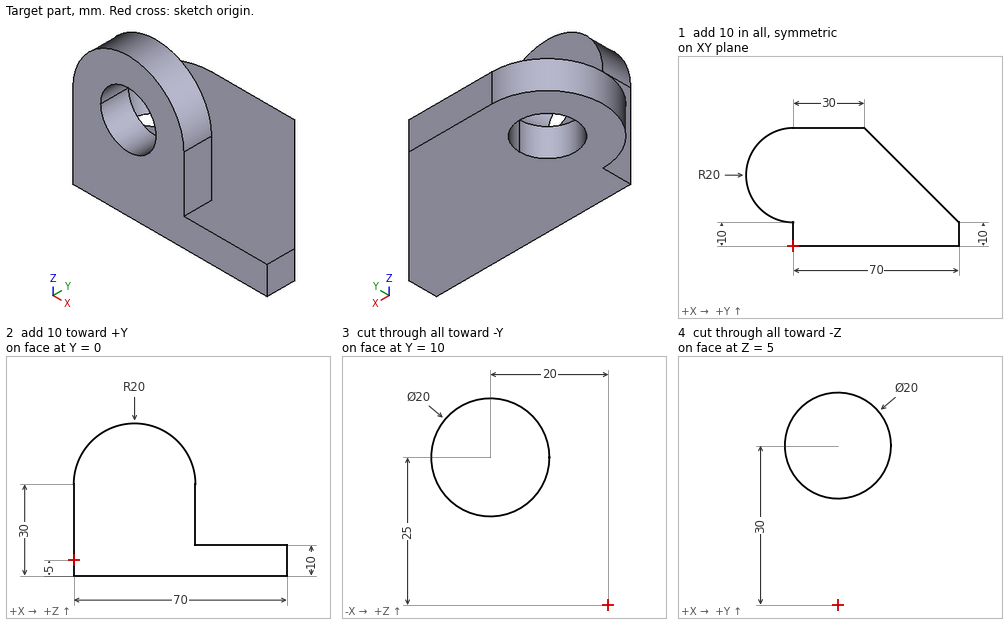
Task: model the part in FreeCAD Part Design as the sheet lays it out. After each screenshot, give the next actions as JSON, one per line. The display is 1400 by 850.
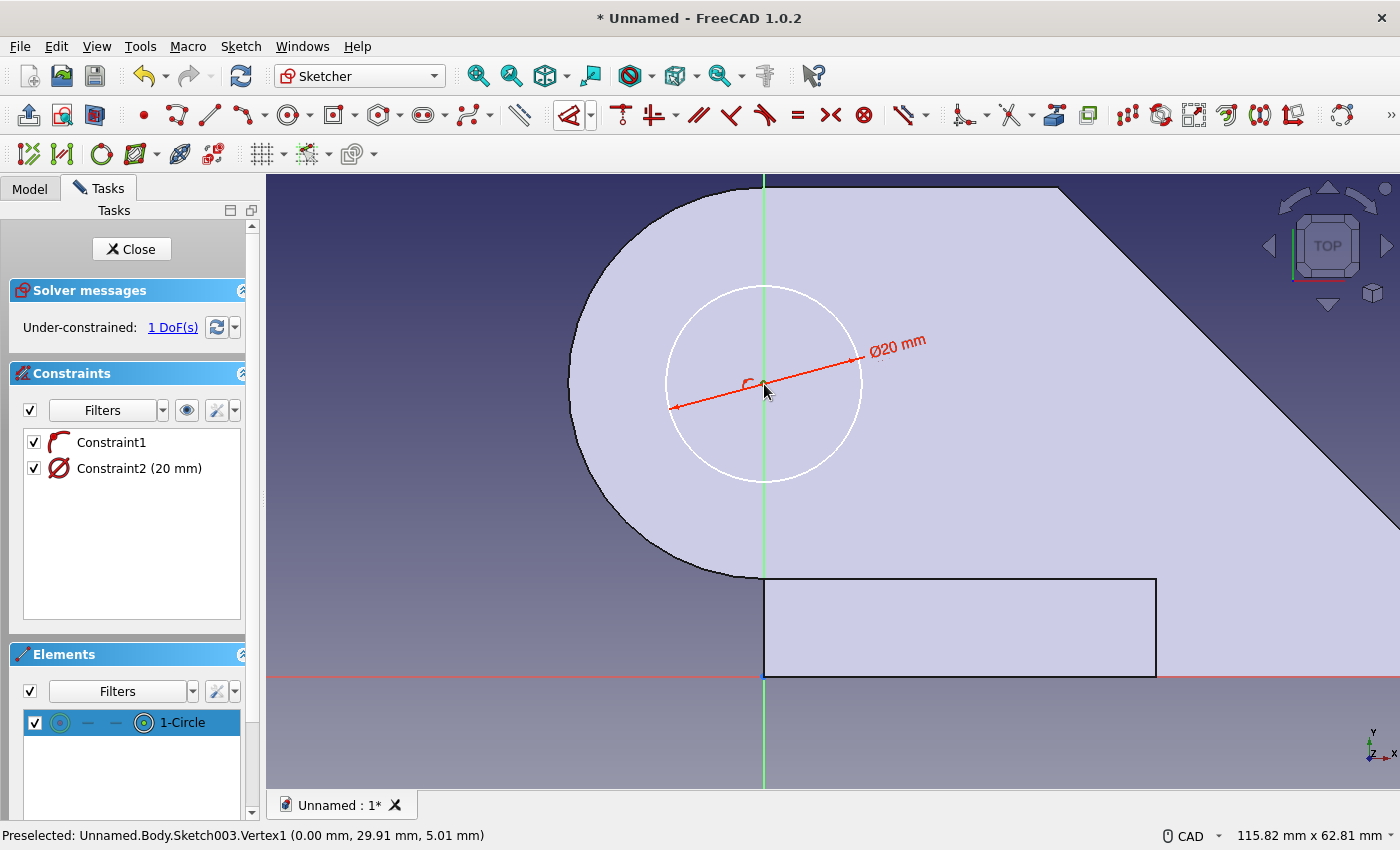
{"action": "left_click", "coordinate": [590, 116]}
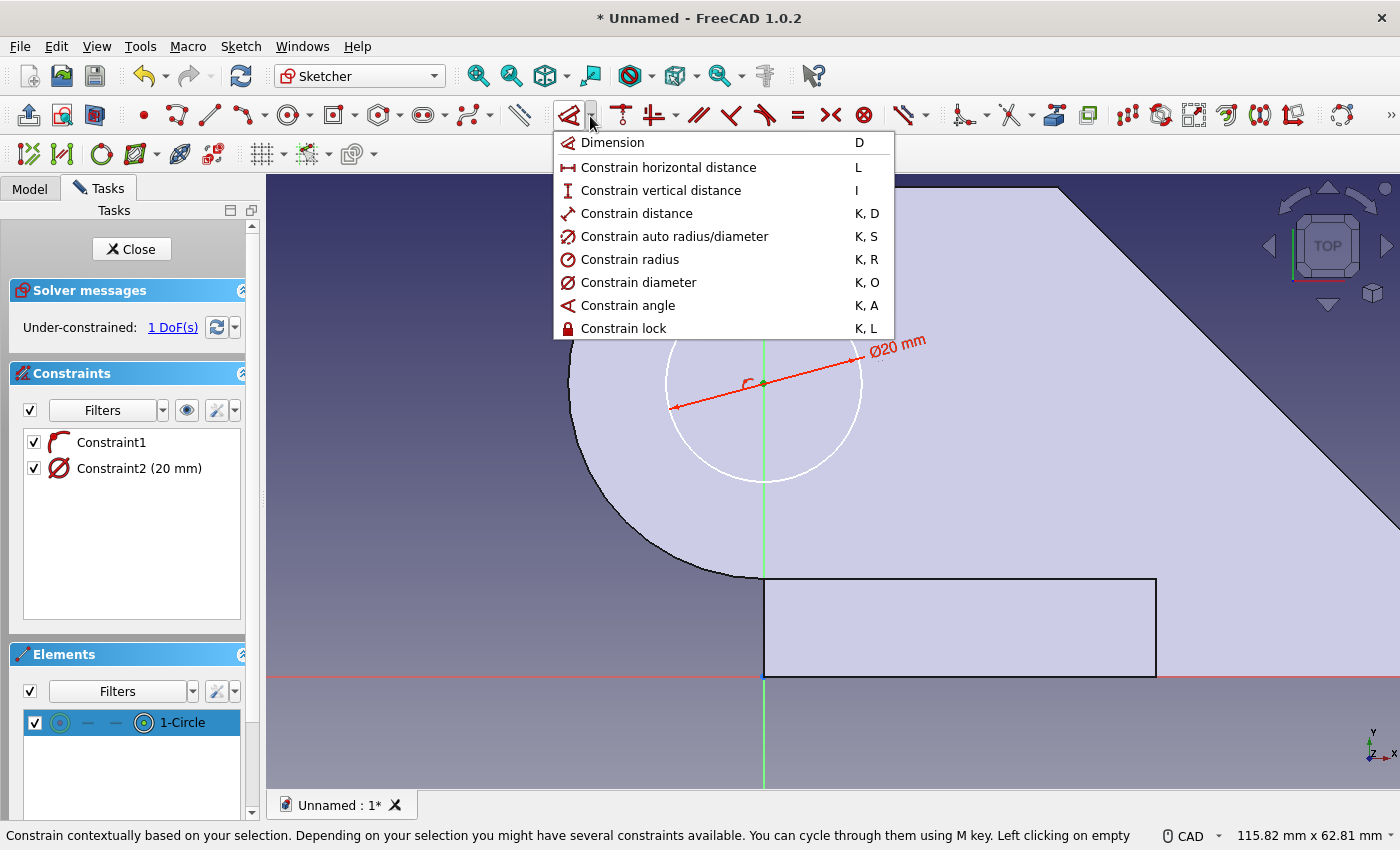
{"action": "left_click", "coordinate": [724, 190]}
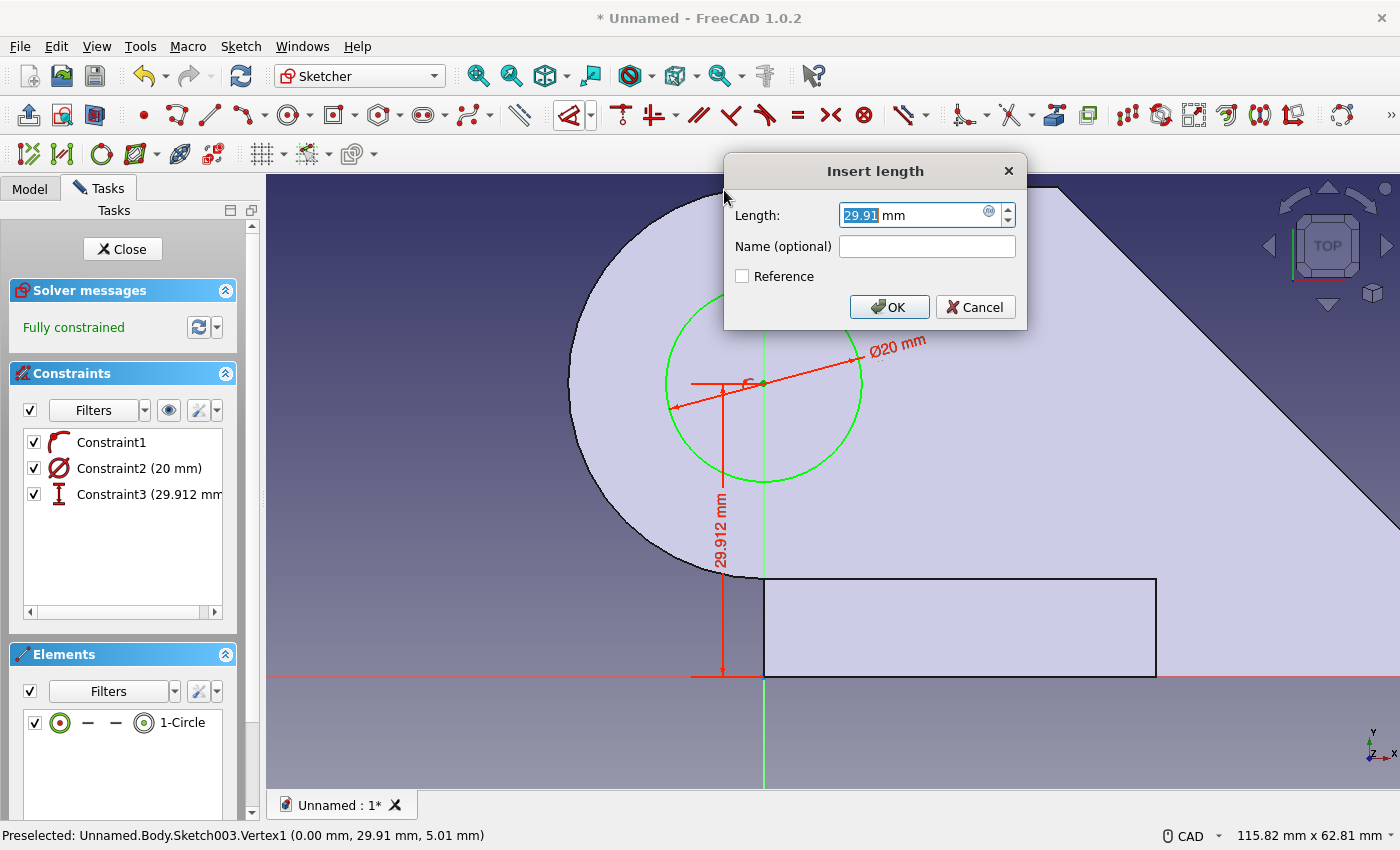
{"action": "type", "text": "30"}
{"action": "key", "text": "Return"}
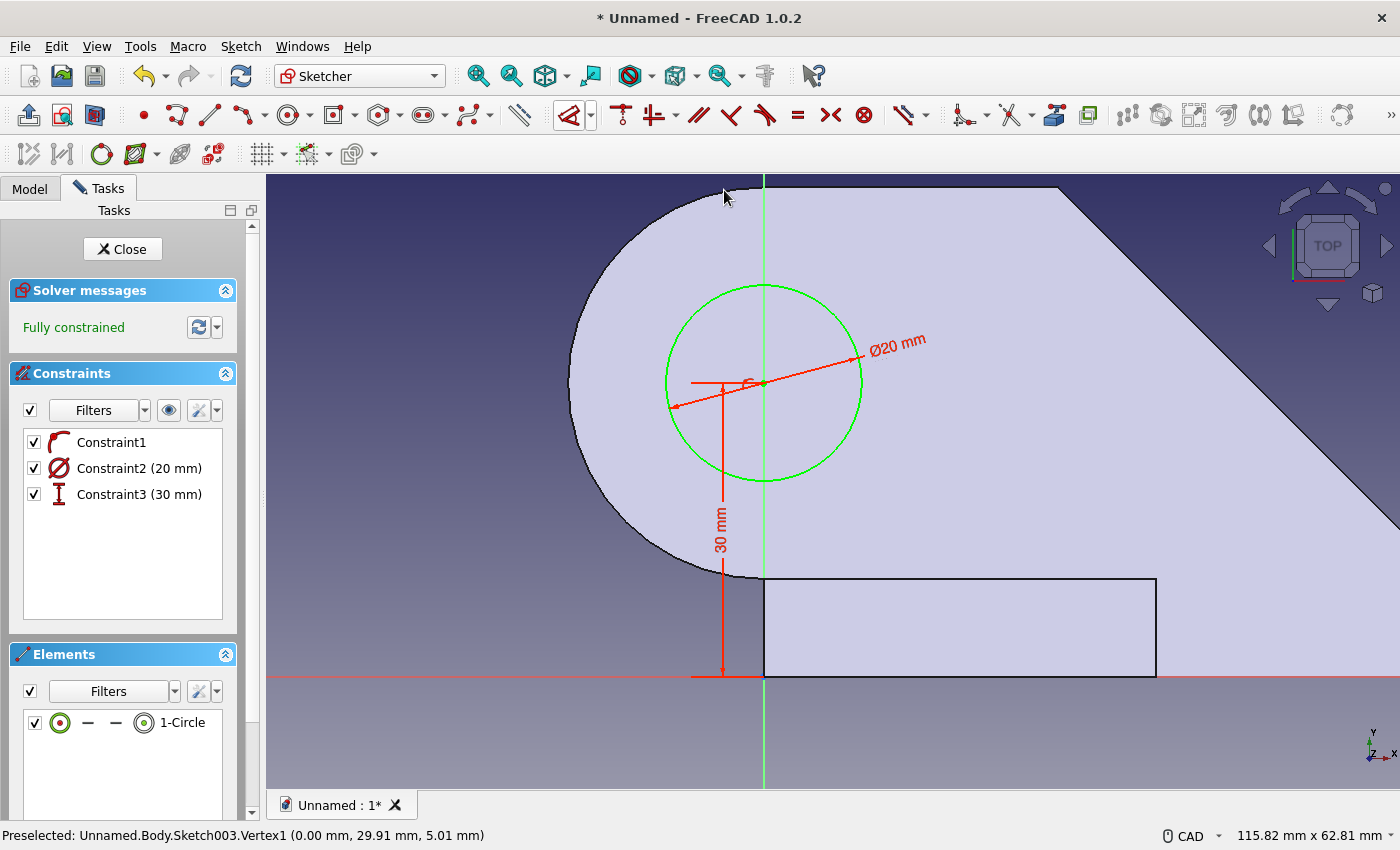
{"action": "left_click", "coordinate": [123, 249]}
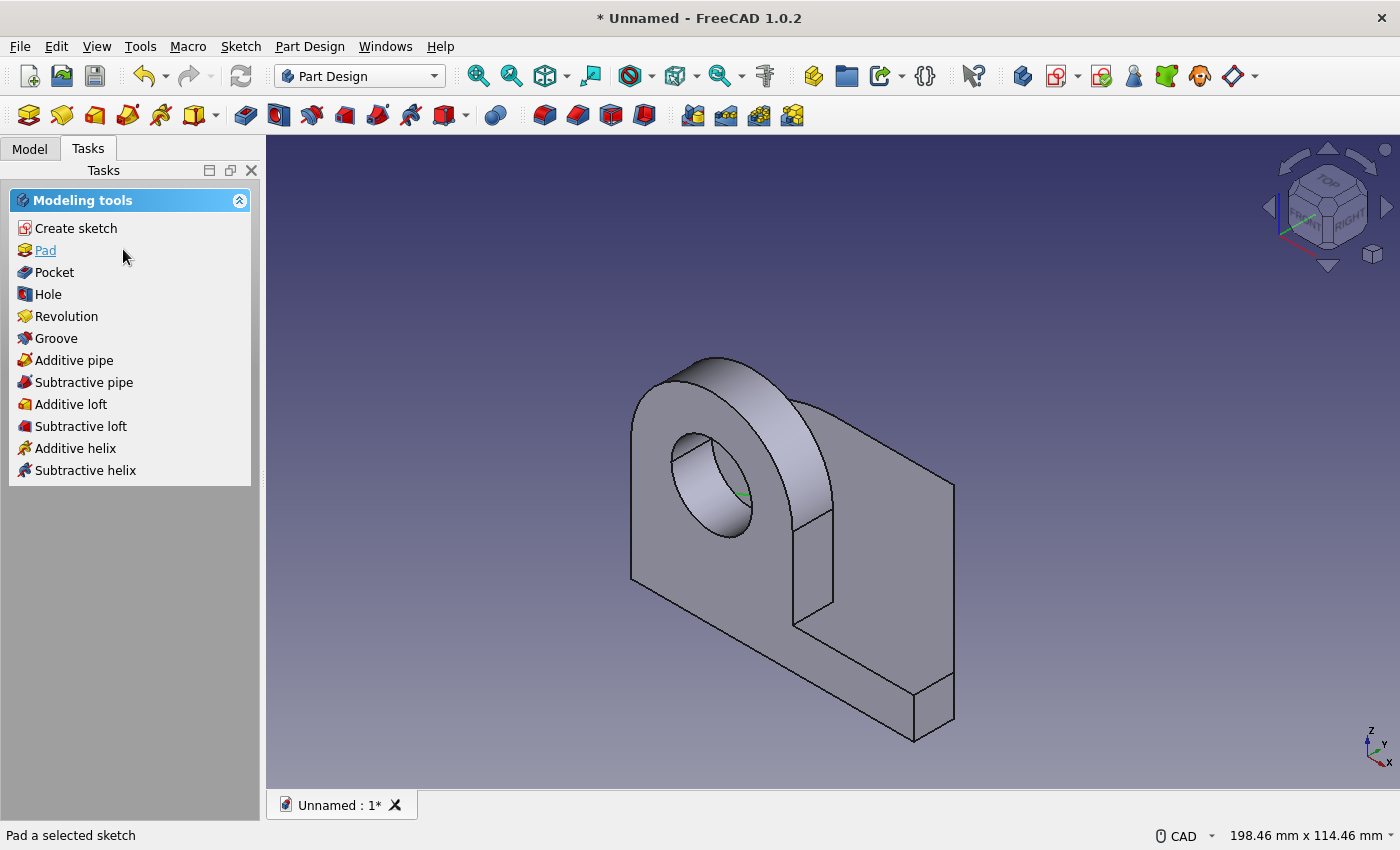
{"action": "left_click", "coordinate": [246, 116]}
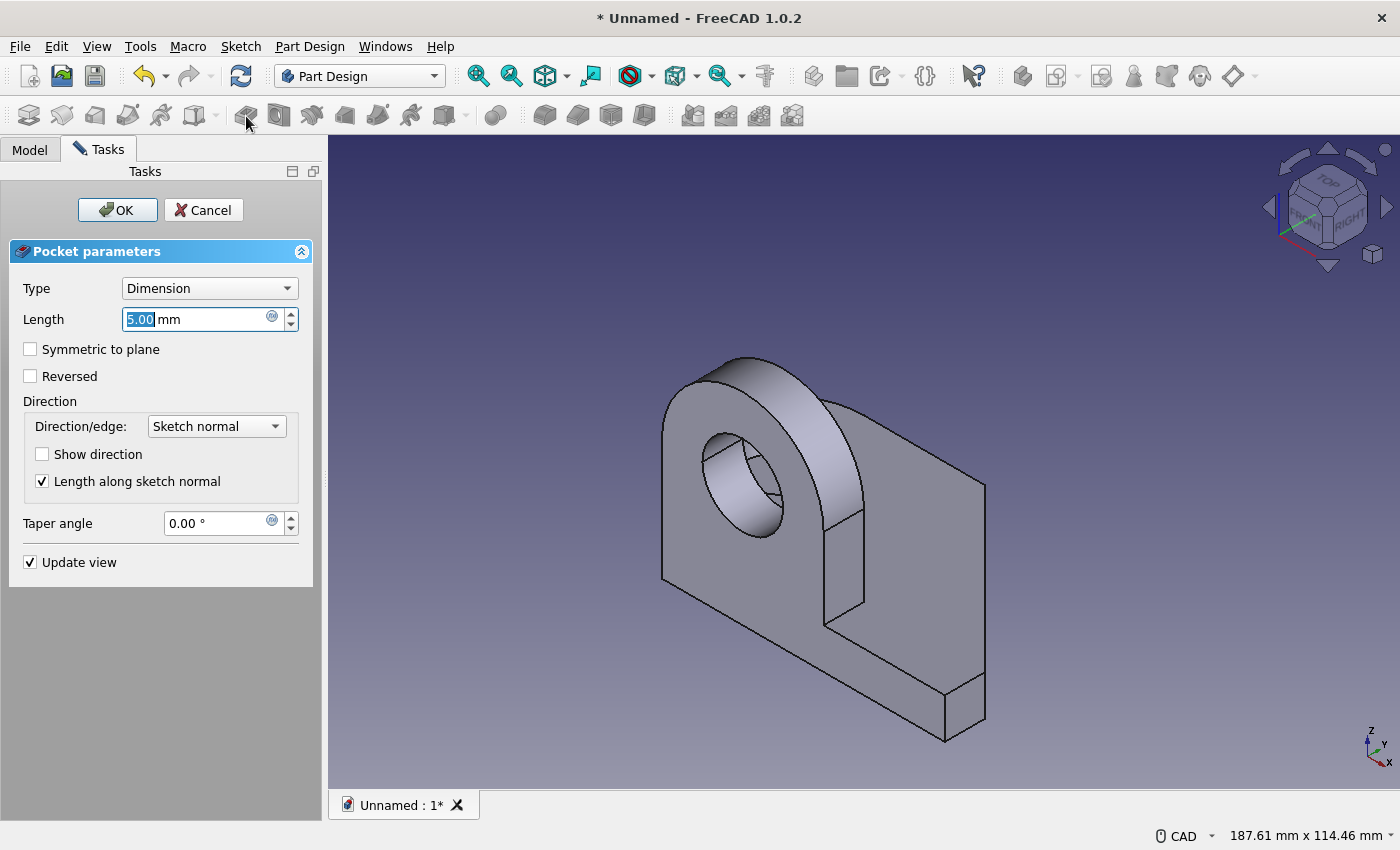
{"action": "left_click", "coordinate": [210, 288]}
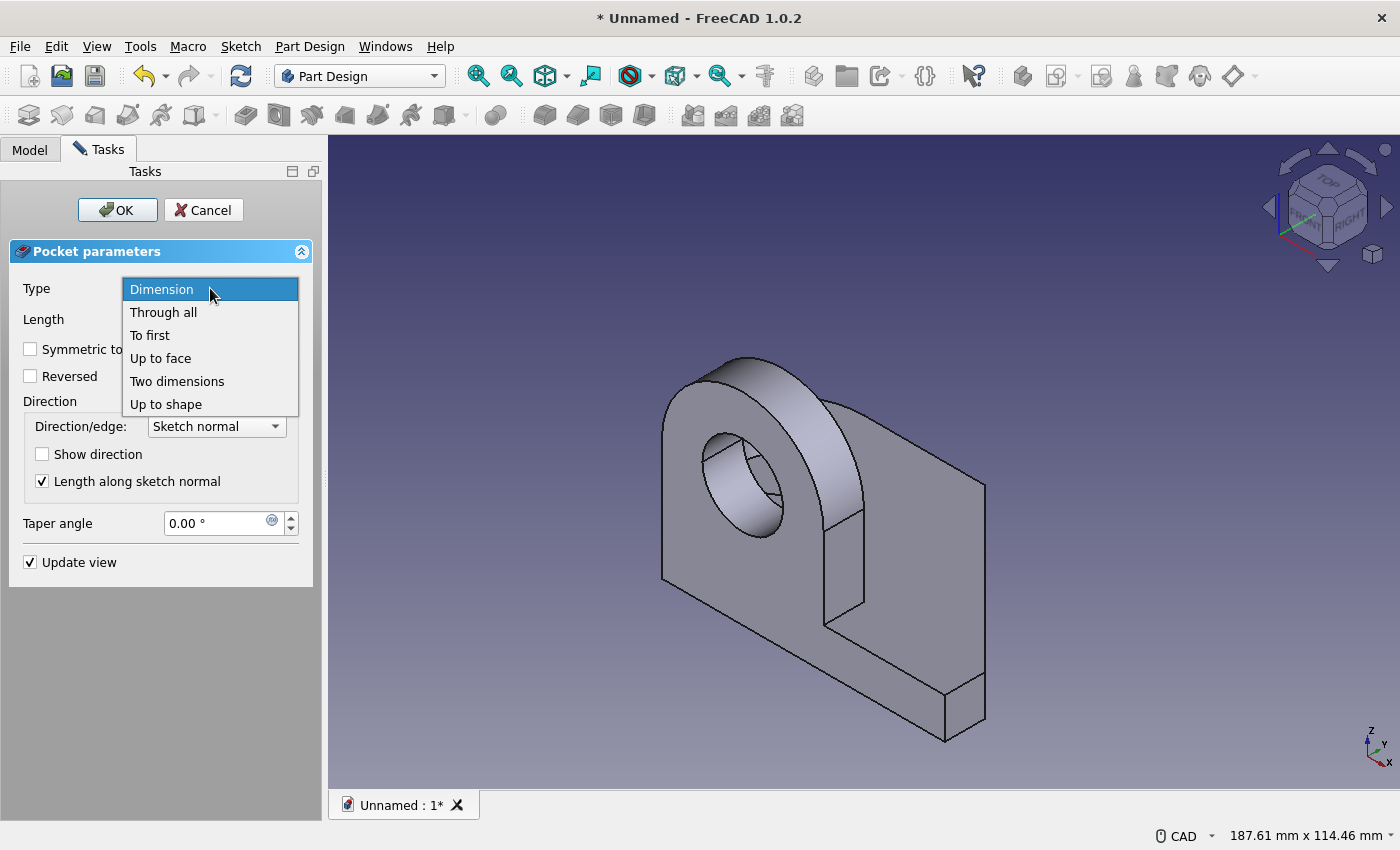
{"action": "left_click", "coordinate": [208, 312]}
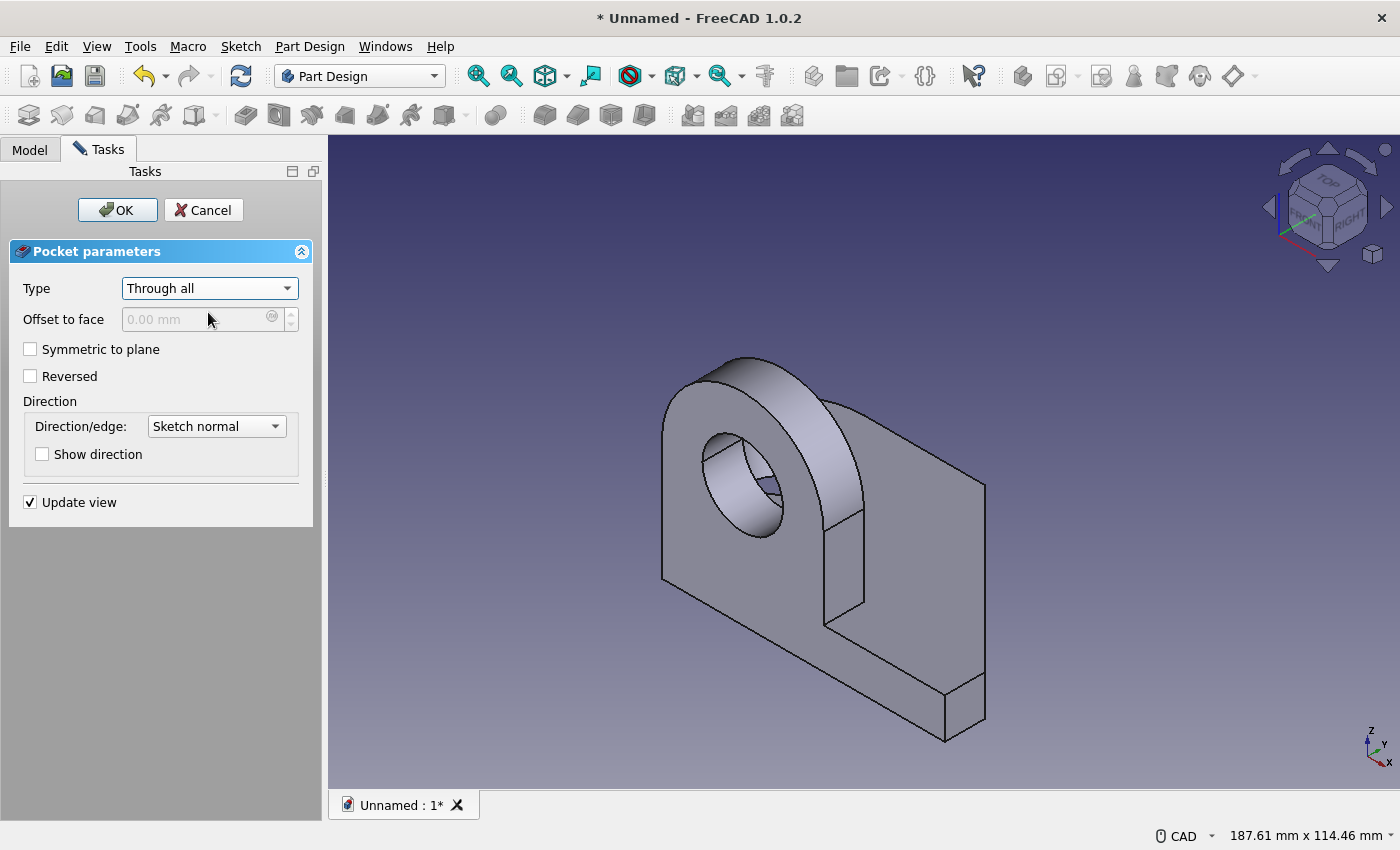
{"action": "left_click", "coordinate": [118, 210]}